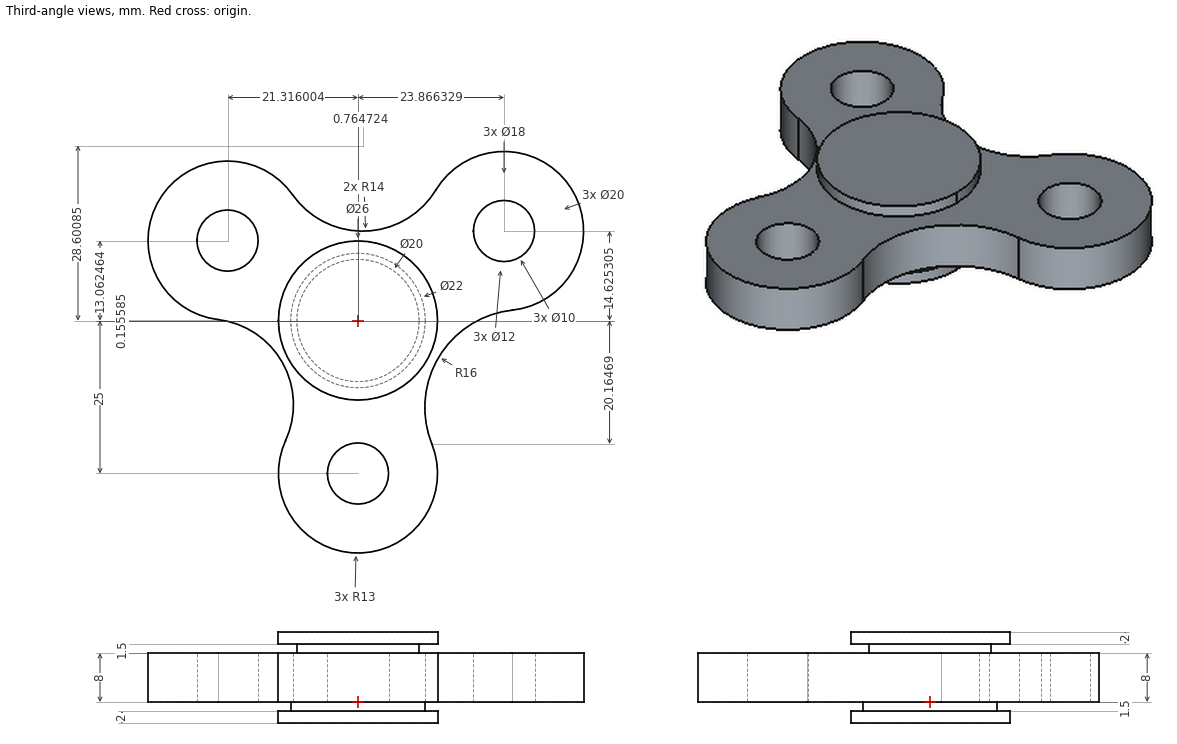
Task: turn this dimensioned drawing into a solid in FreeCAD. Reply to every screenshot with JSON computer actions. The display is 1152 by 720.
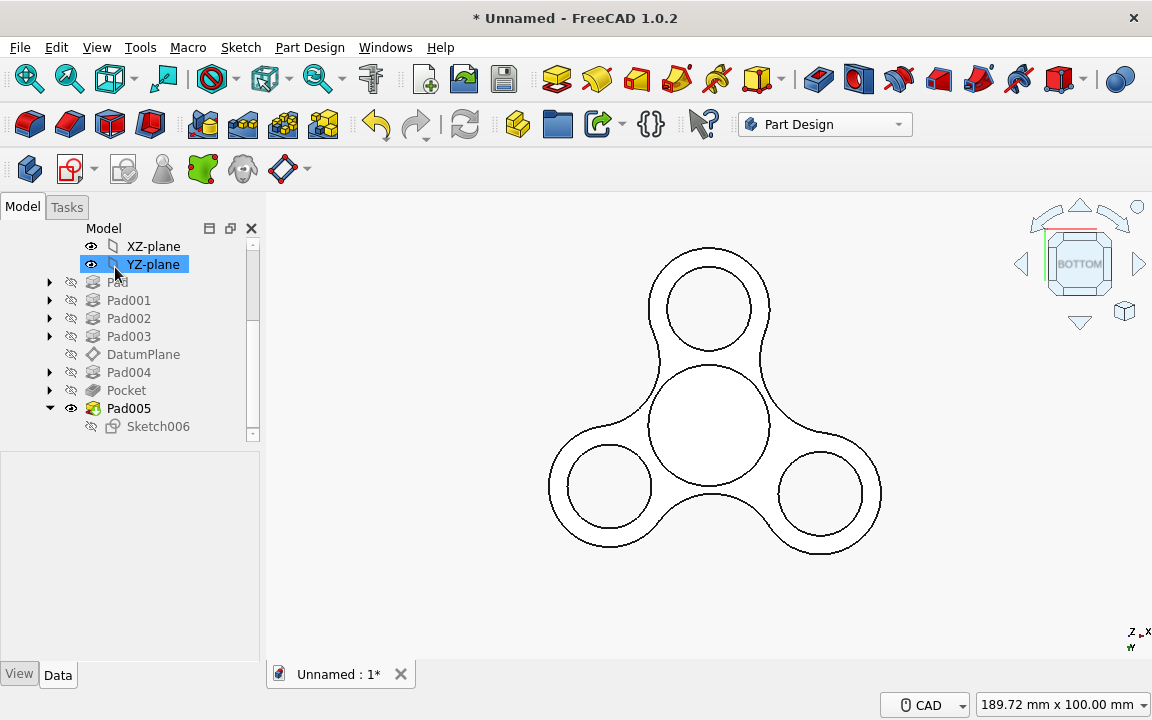
{"action": "left_click", "coordinate": [762, 488]}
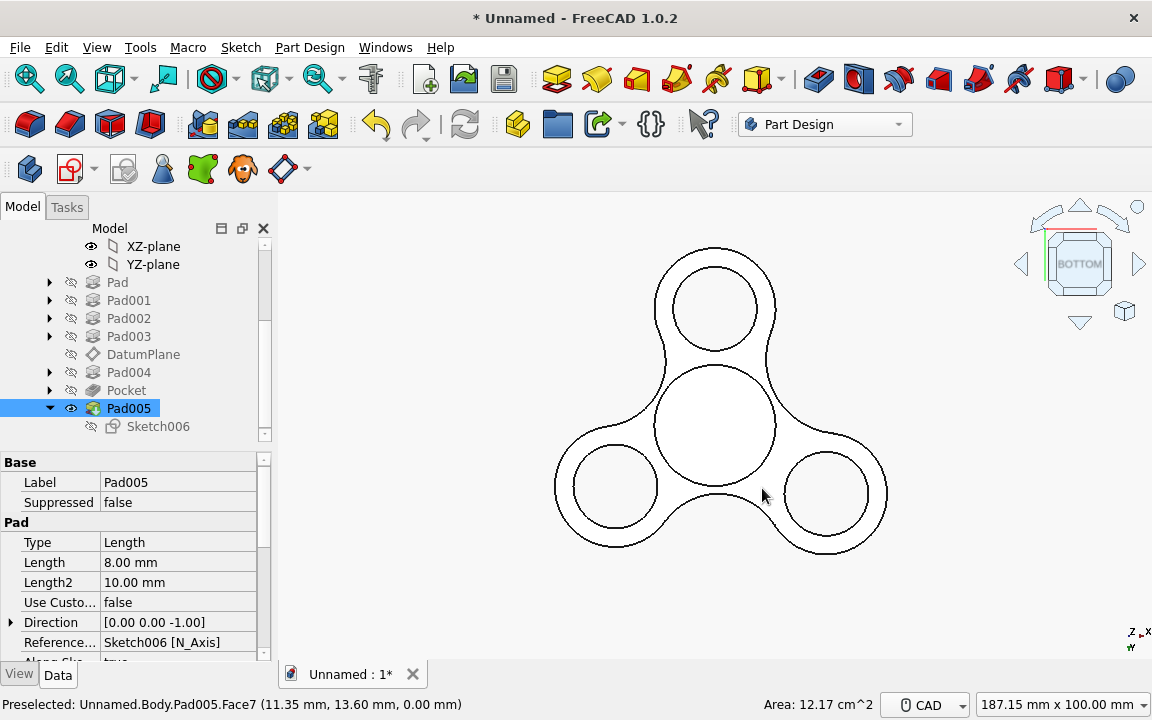
{"action": "left_click", "coordinate": [70, 170]}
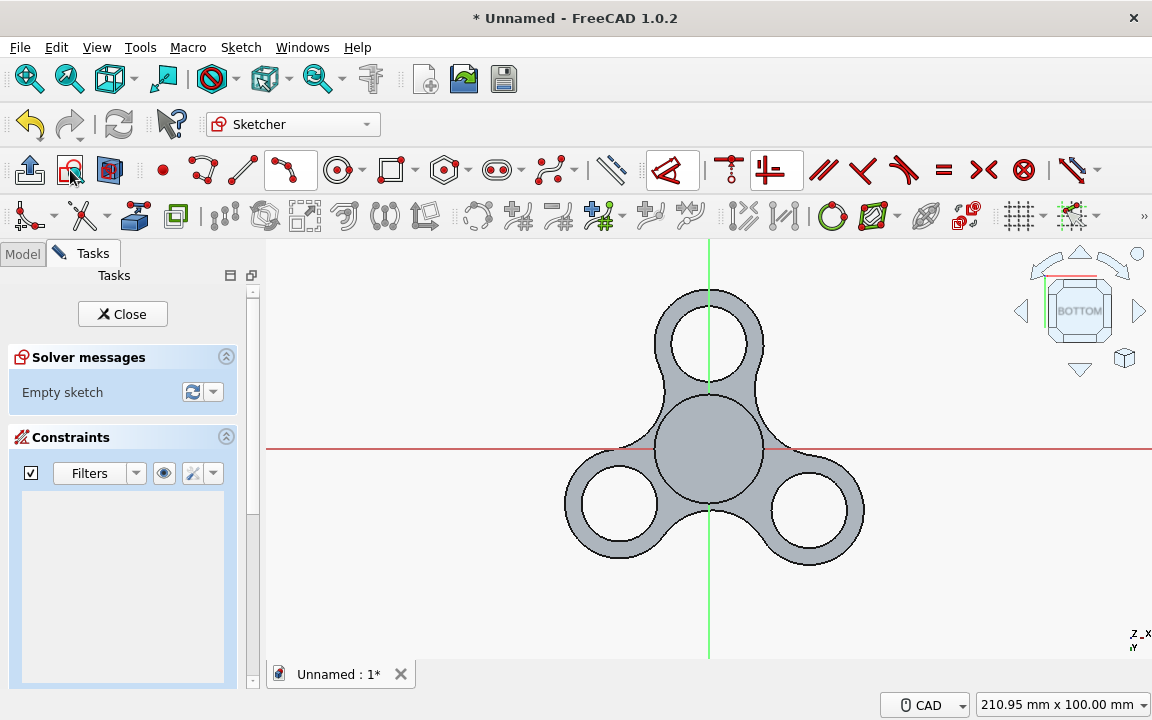
{"action": "left_click", "coordinate": [110, 170]}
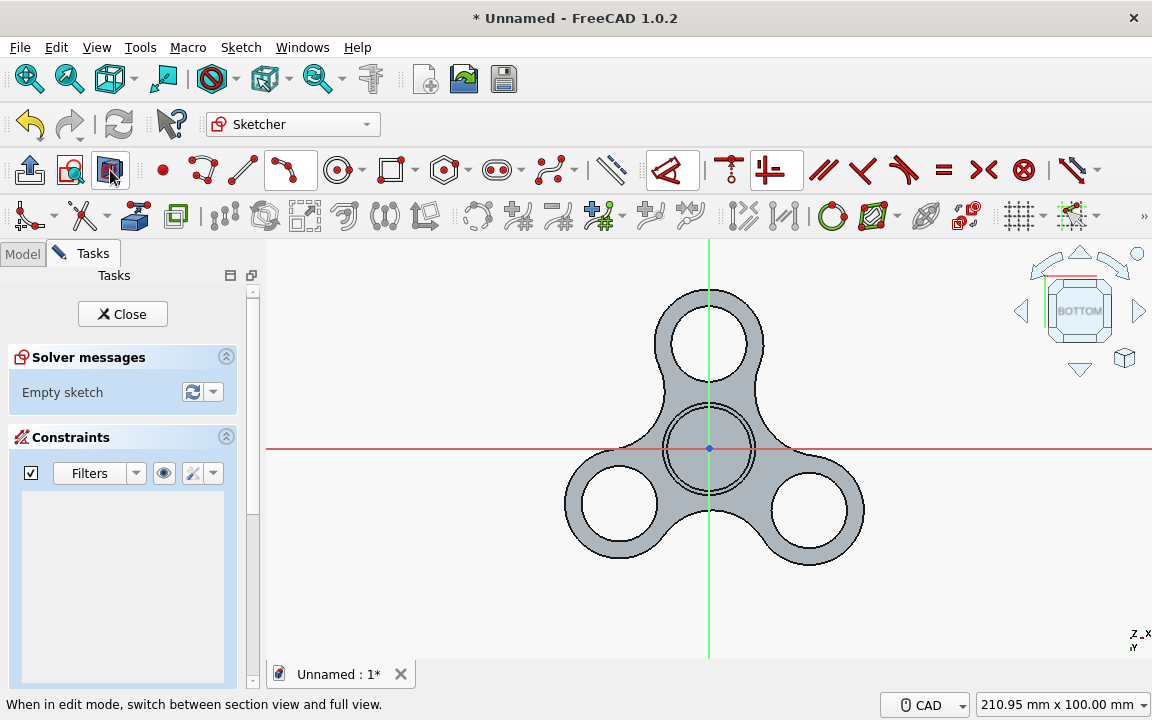
{"action": "left_click", "coordinate": [338, 170]}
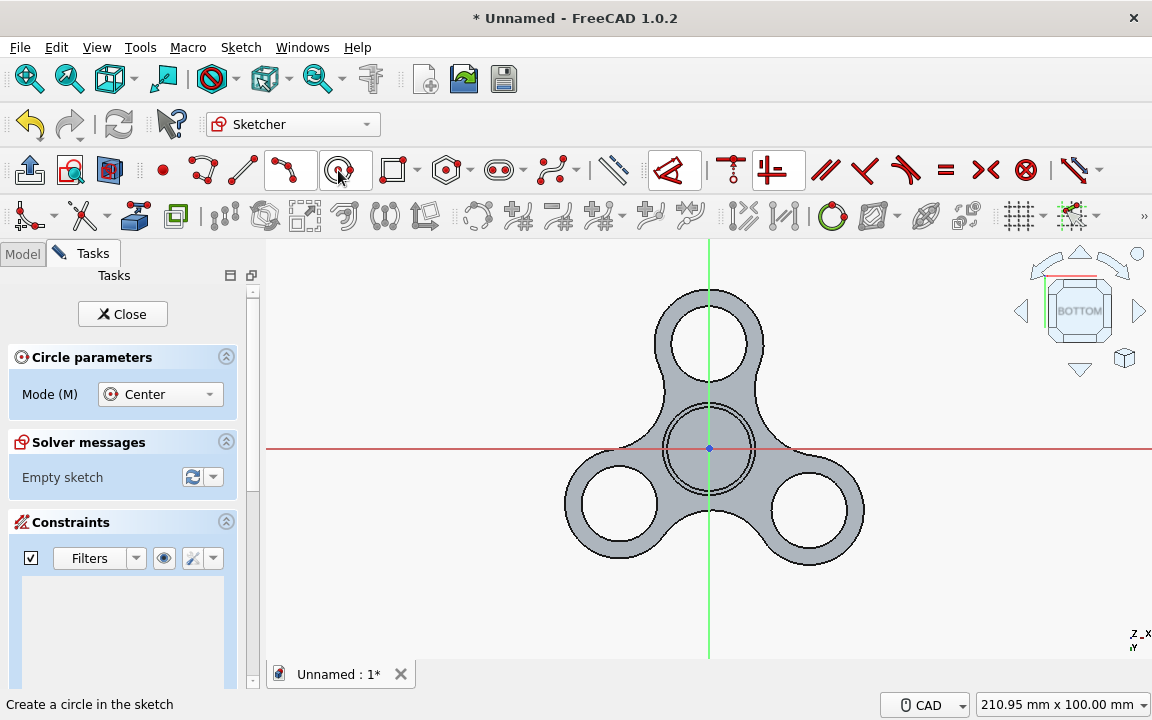
{"action": "left_click", "coordinate": [809, 510]}
{"action": "mouse_move", "coordinate": [836, 484]}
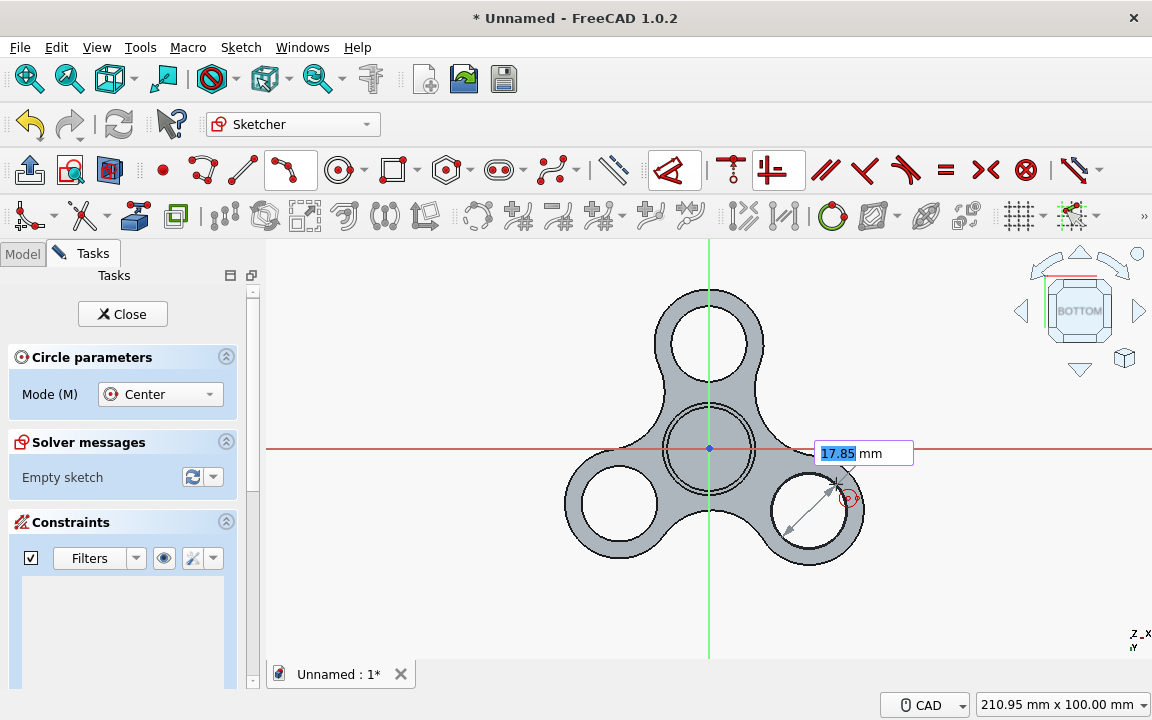
{"action": "type", "text": "18"}
{"action": "key", "text": "Return"}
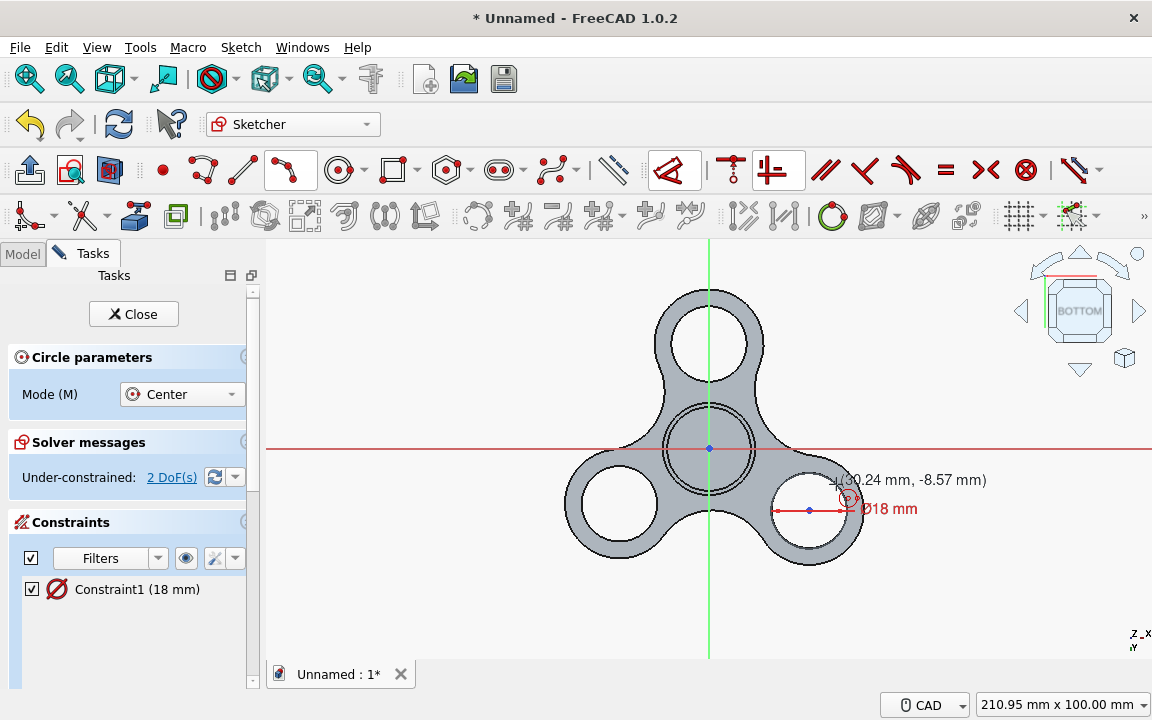
{"action": "left_click", "coordinate": [619, 504]}
{"action": "mouse_move", "coordinate": [646, 477]}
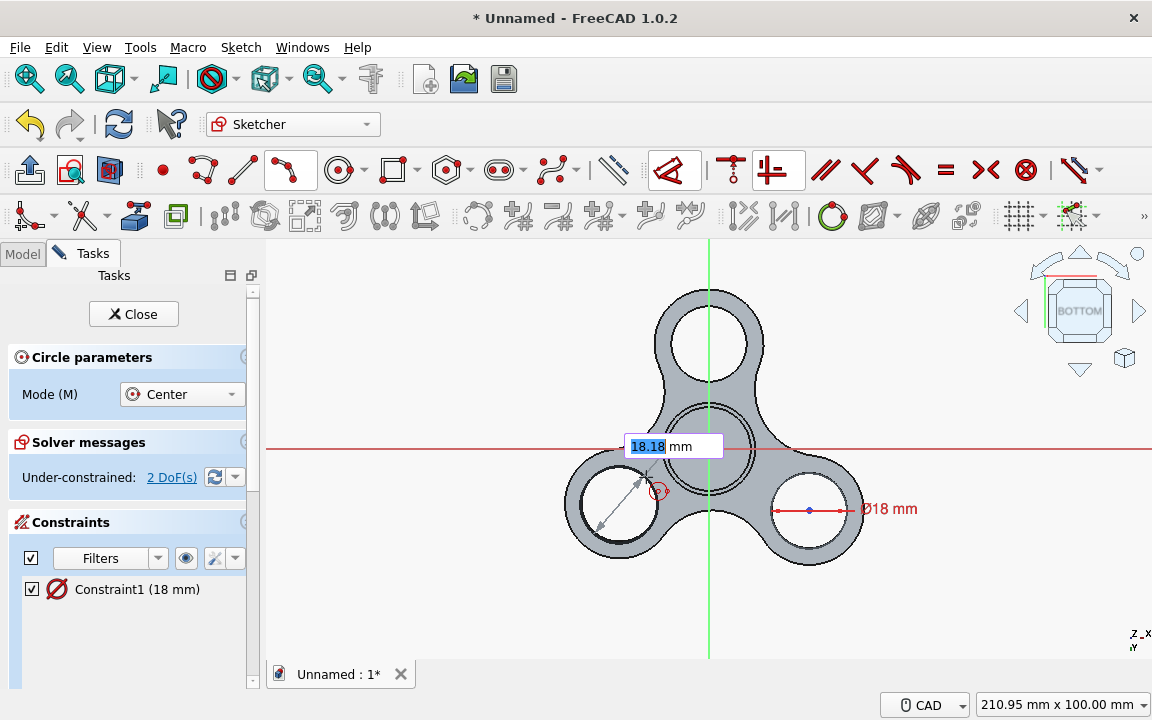
{"action": "type", "text": "18"}
{"action": "key", "text": "Return"}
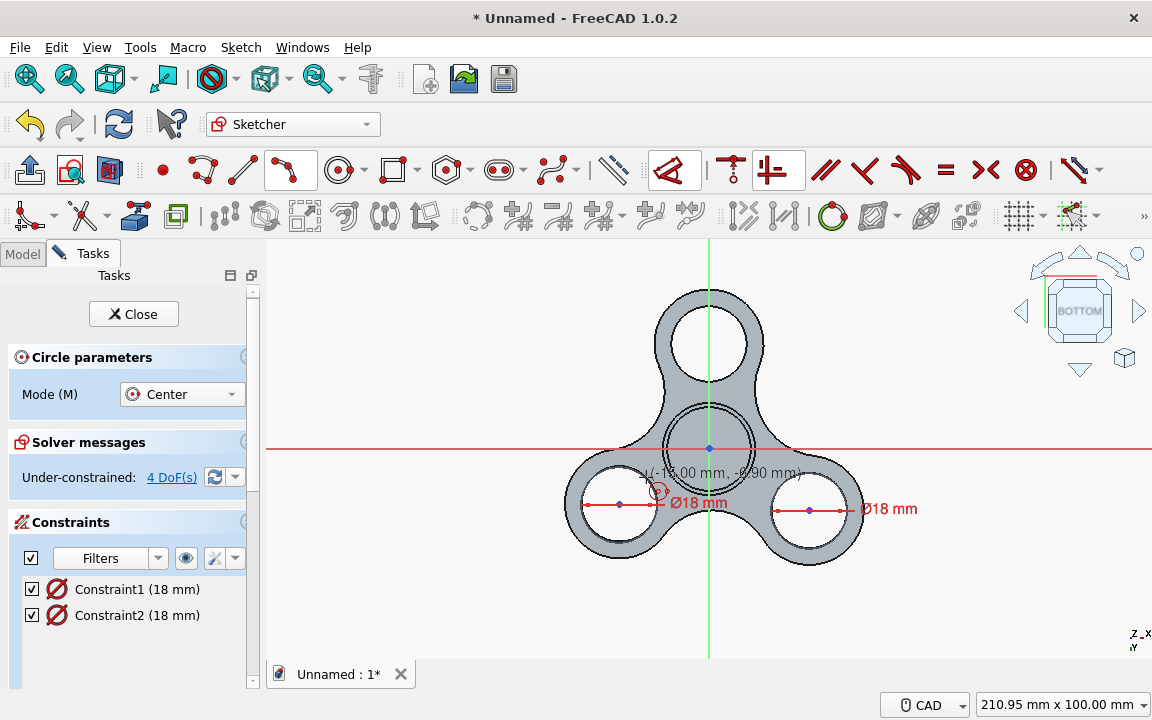
{"action": "left_click", "coordinate": [709, 344]}
{"action": "mouse_move", "coordinate": [736, 317]}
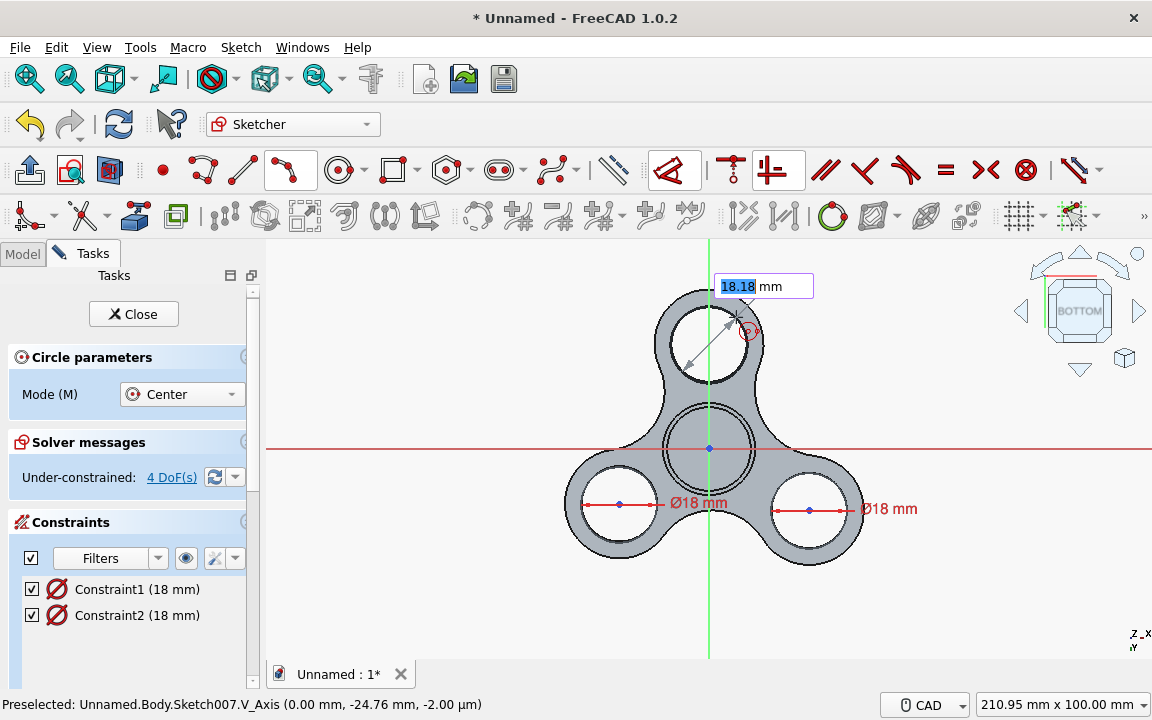
{"action": "type", "text": "18"}
{"action": "key", "text": "Return"}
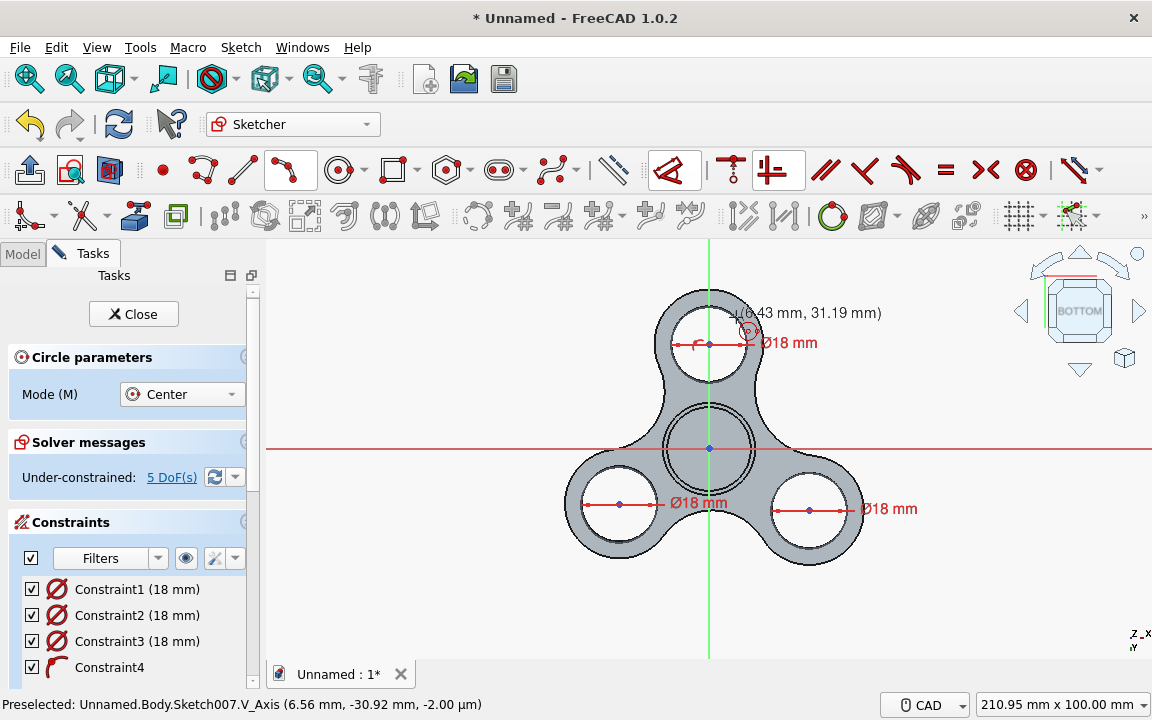
{"action": "left_click", "coordinate": [809, 511]}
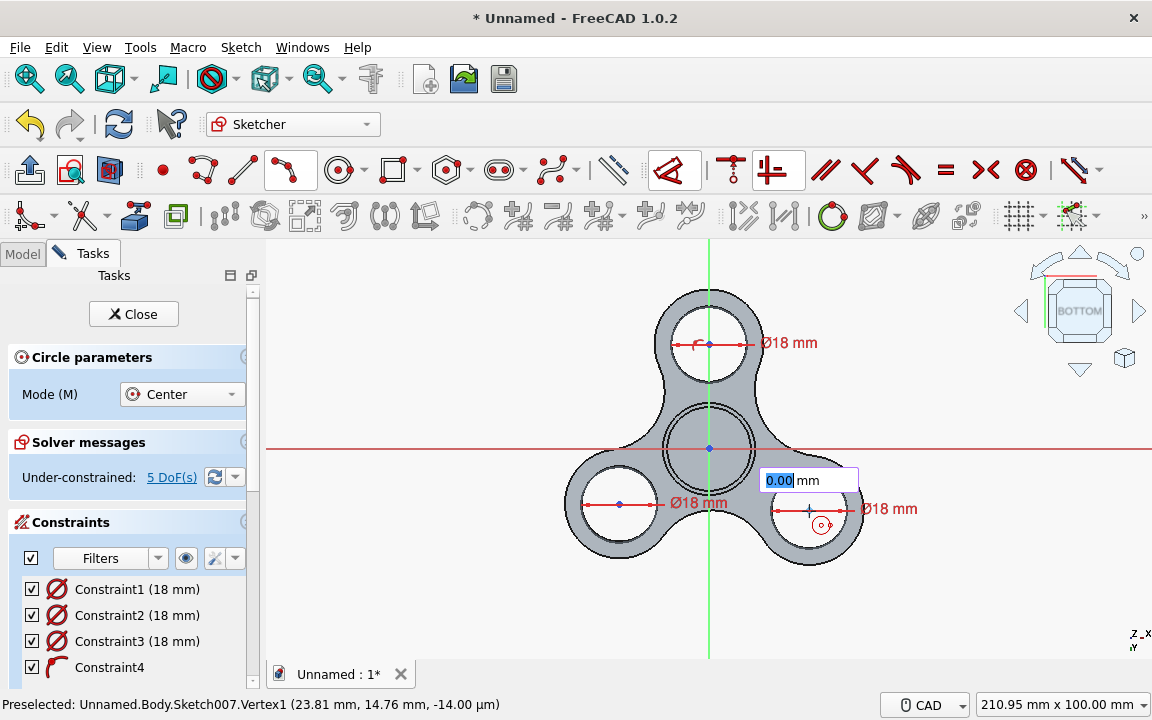
{"action": "scroll", "coordinate": [827, 493], "scroll_direction": "up", "scroll_amount": 2}
{"action": "mouse_move", "coordinate": [827, 492]}